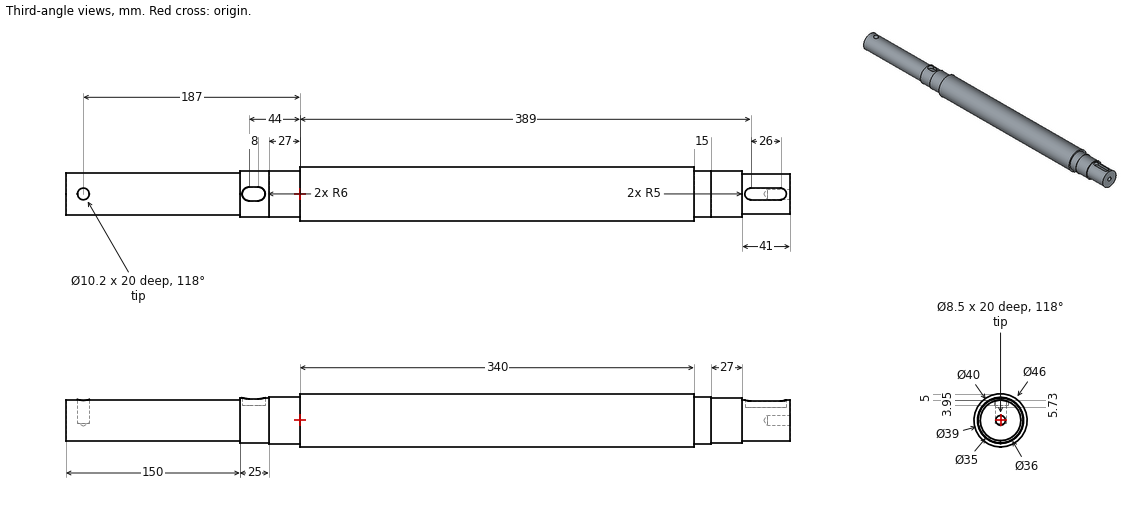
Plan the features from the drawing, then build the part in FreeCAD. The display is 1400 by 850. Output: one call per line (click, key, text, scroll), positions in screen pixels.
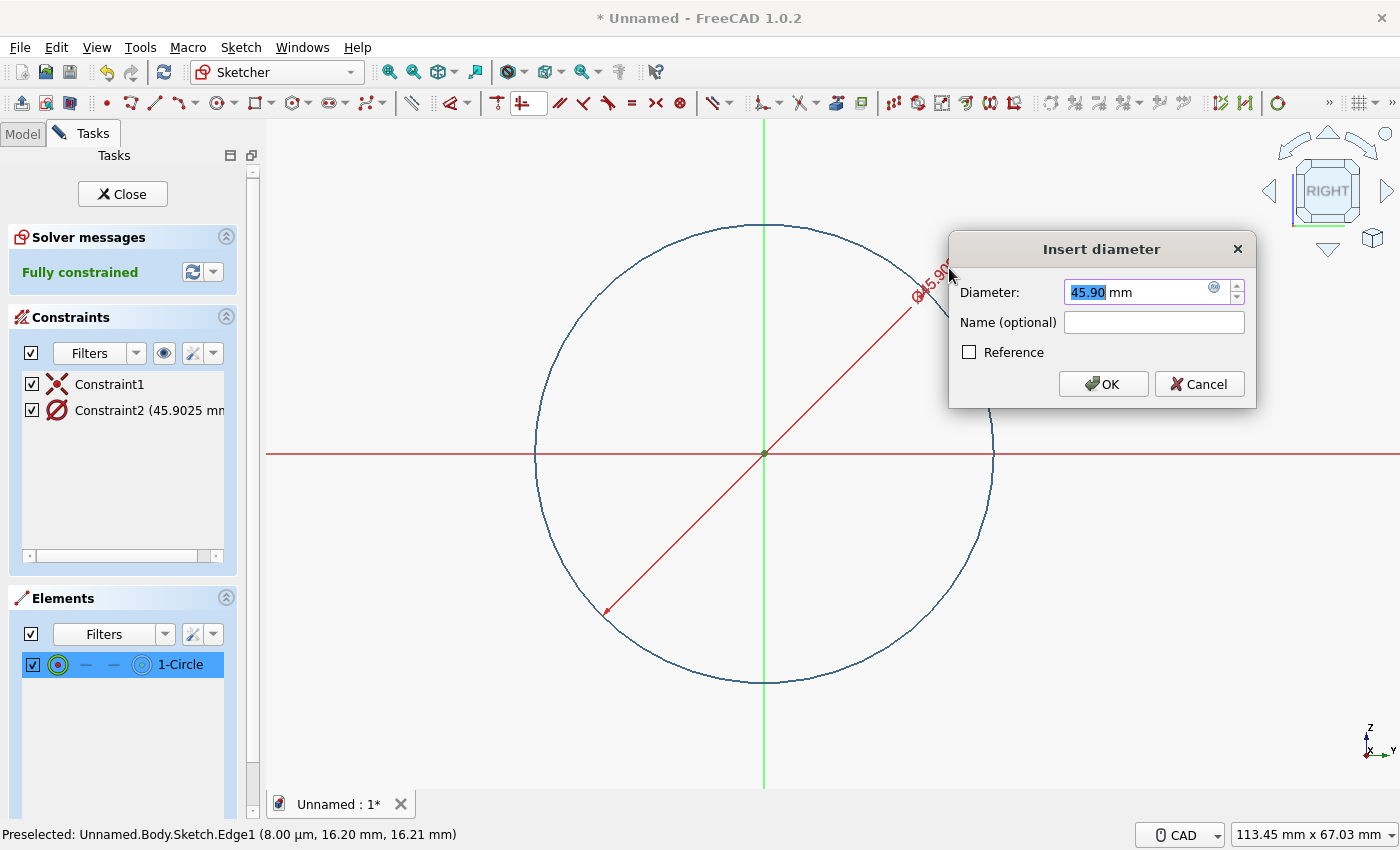
text(46)
key(Return)
key(Escape)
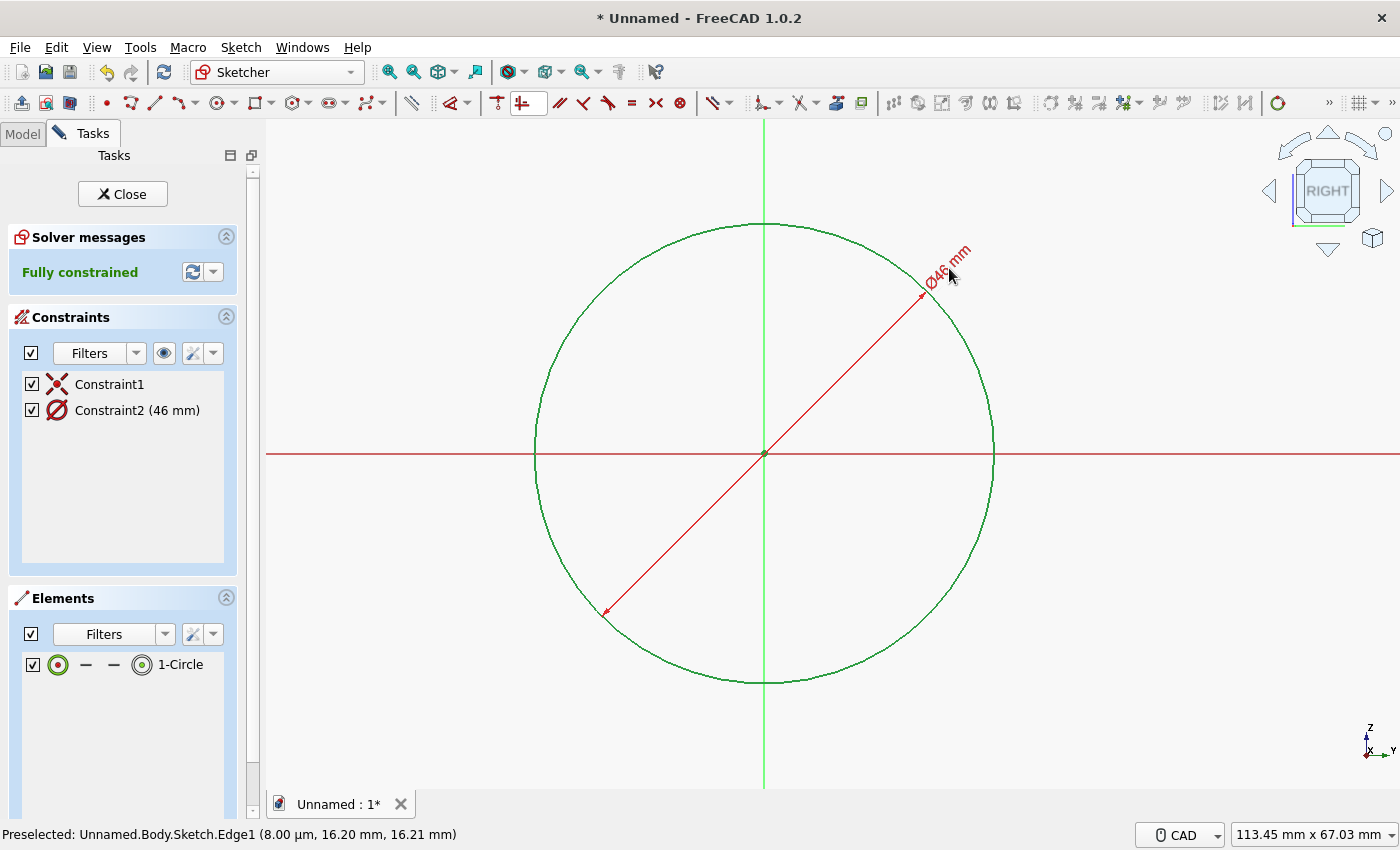
click(123, 194)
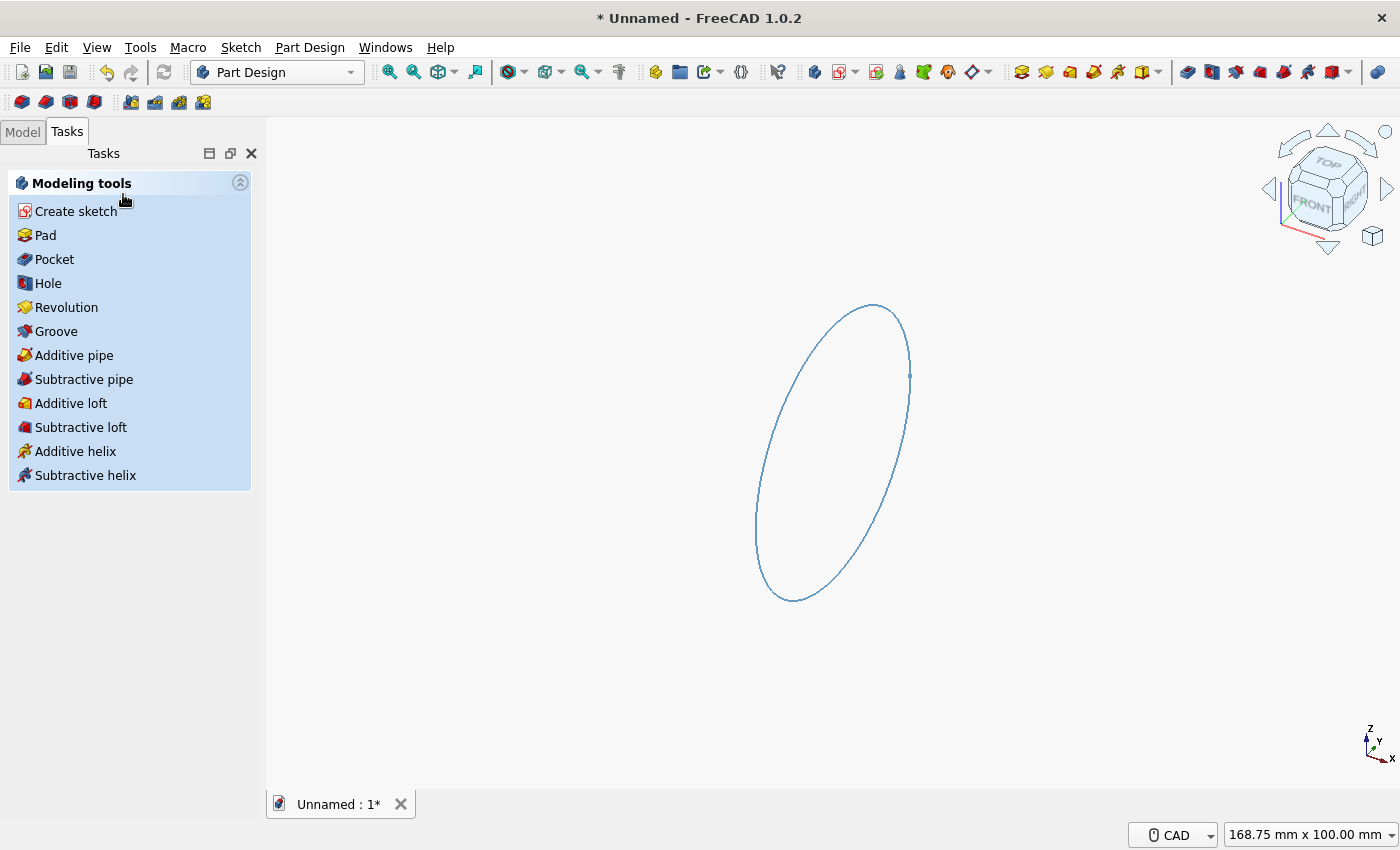
click(1022, 72)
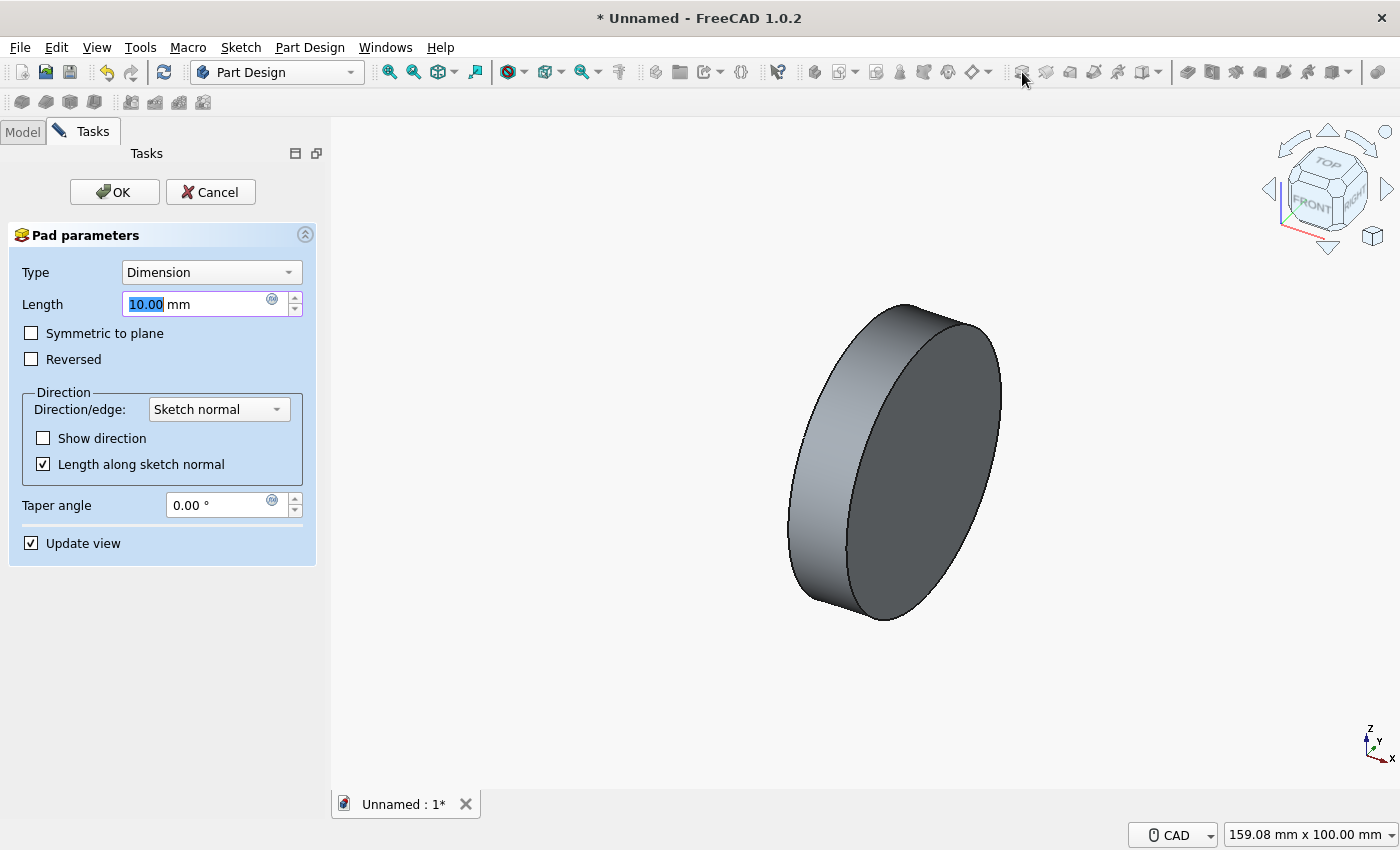
text(340)
key(Tab)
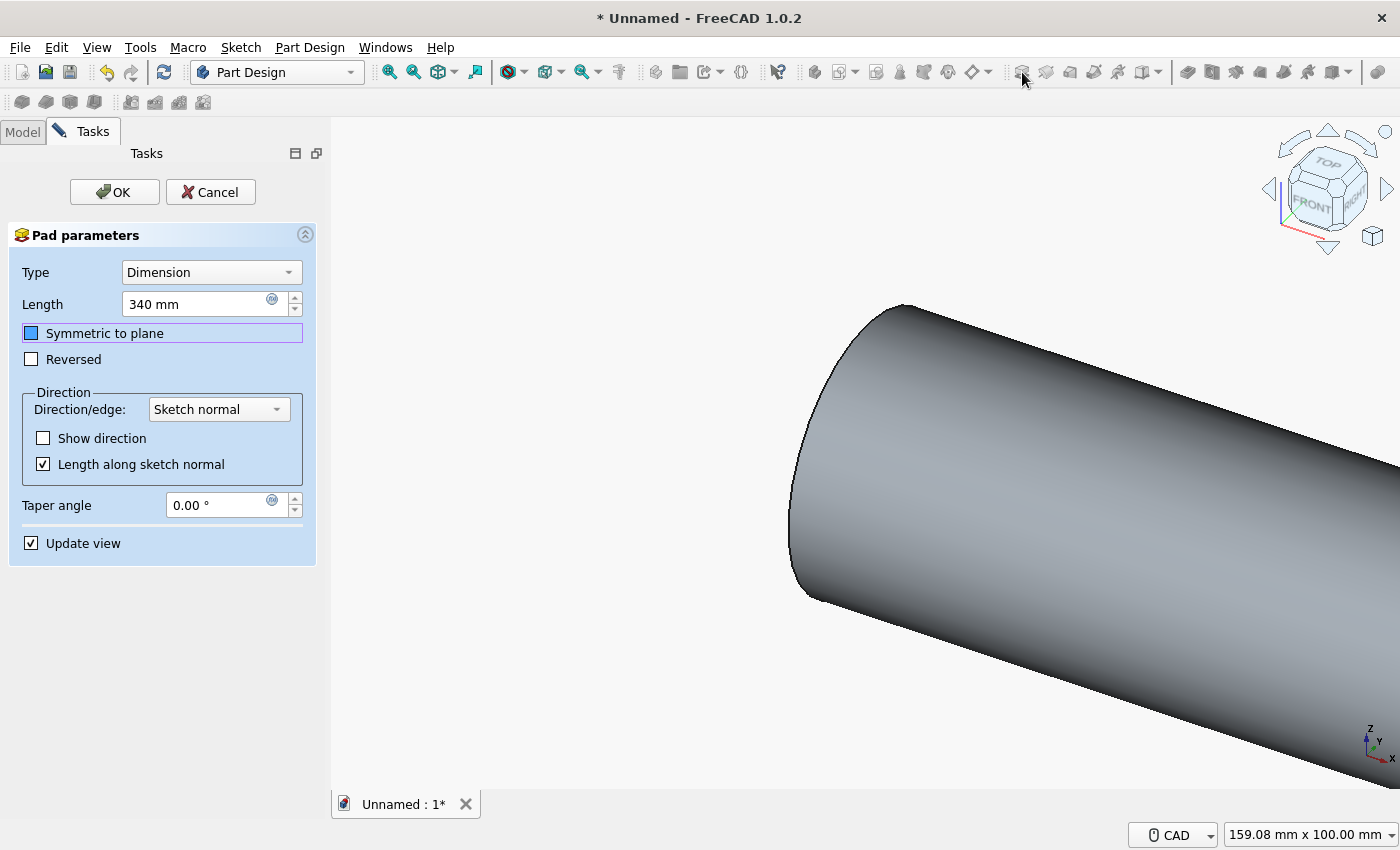
click(115, 192)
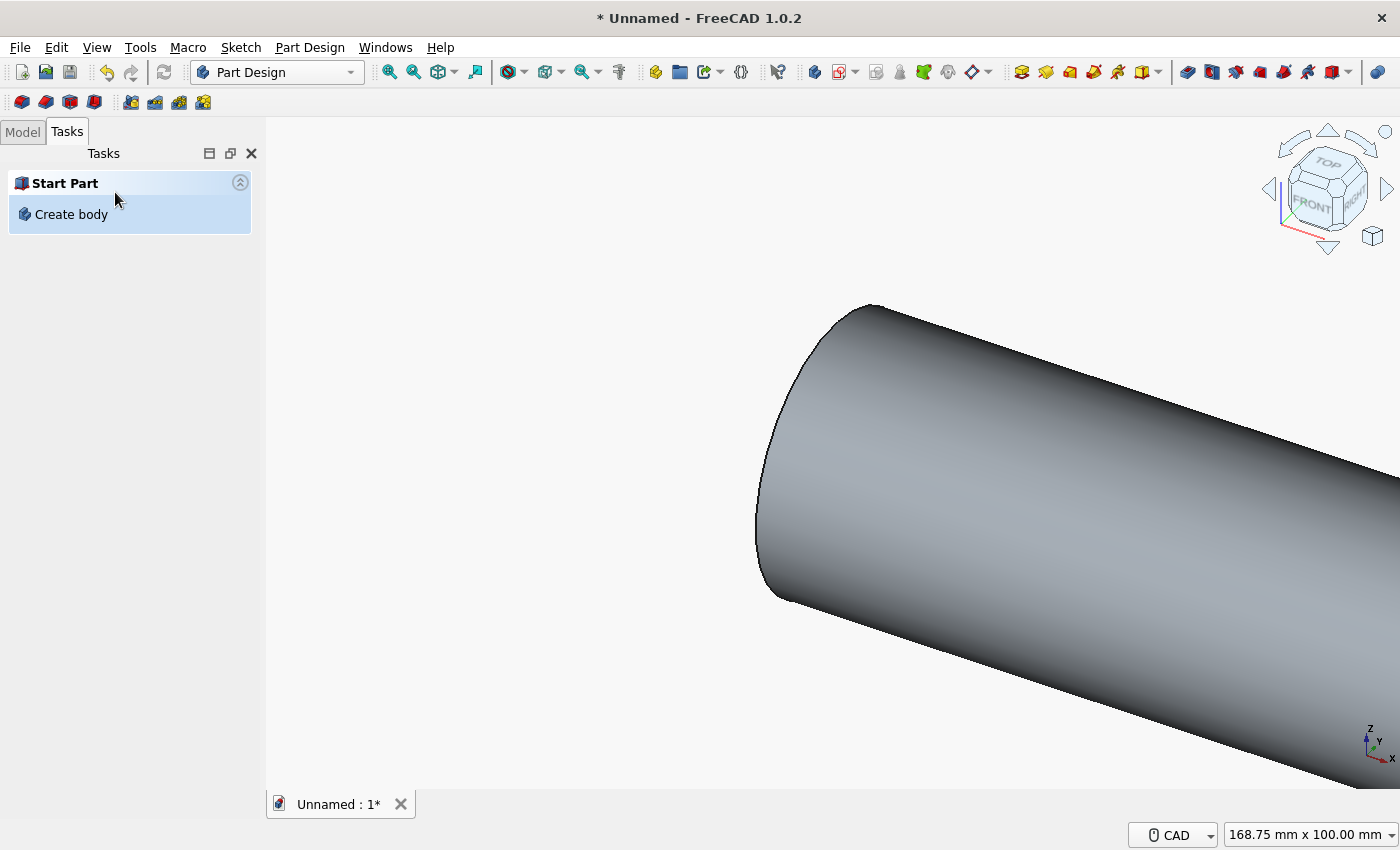
click(390, 72)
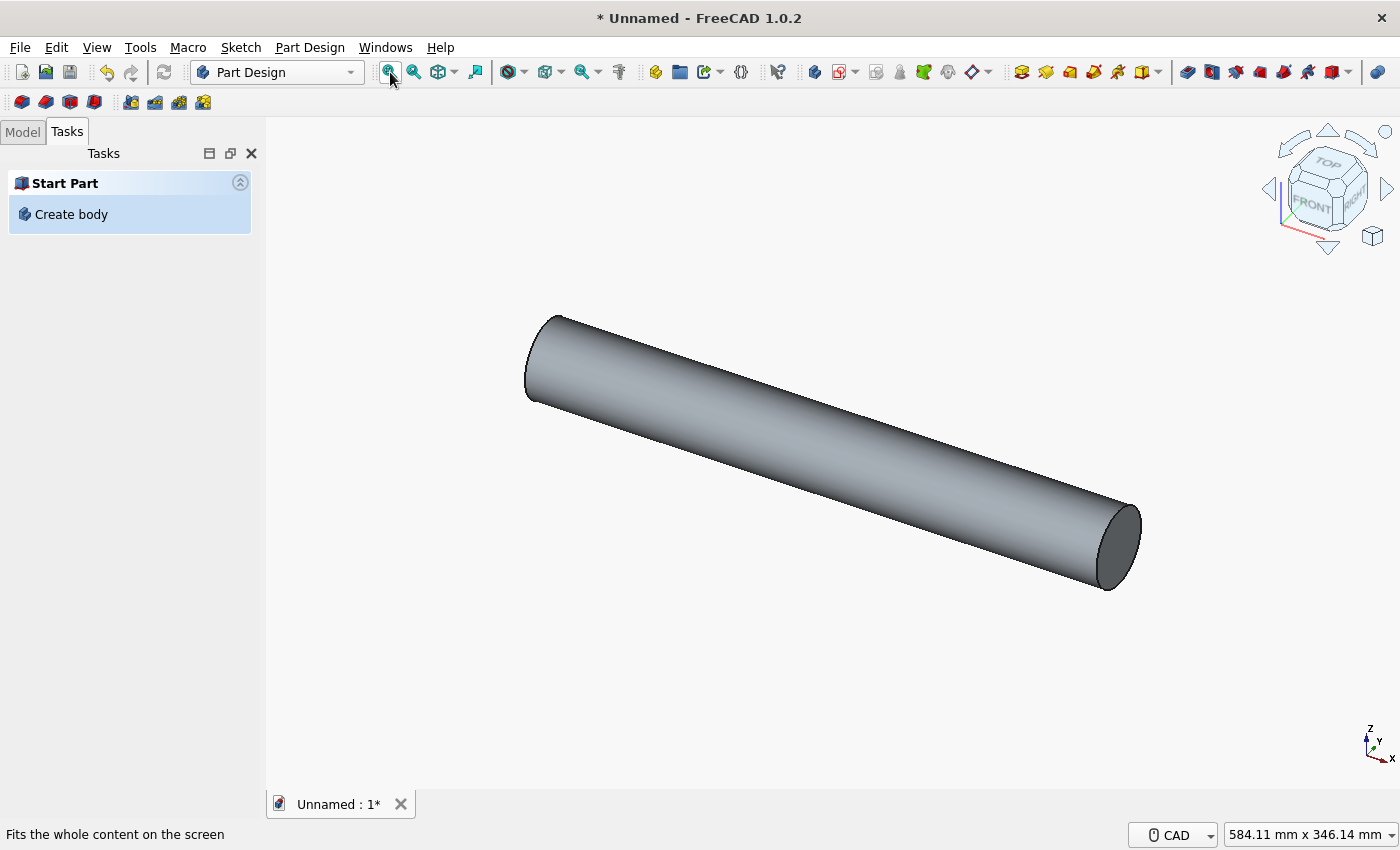
key(6)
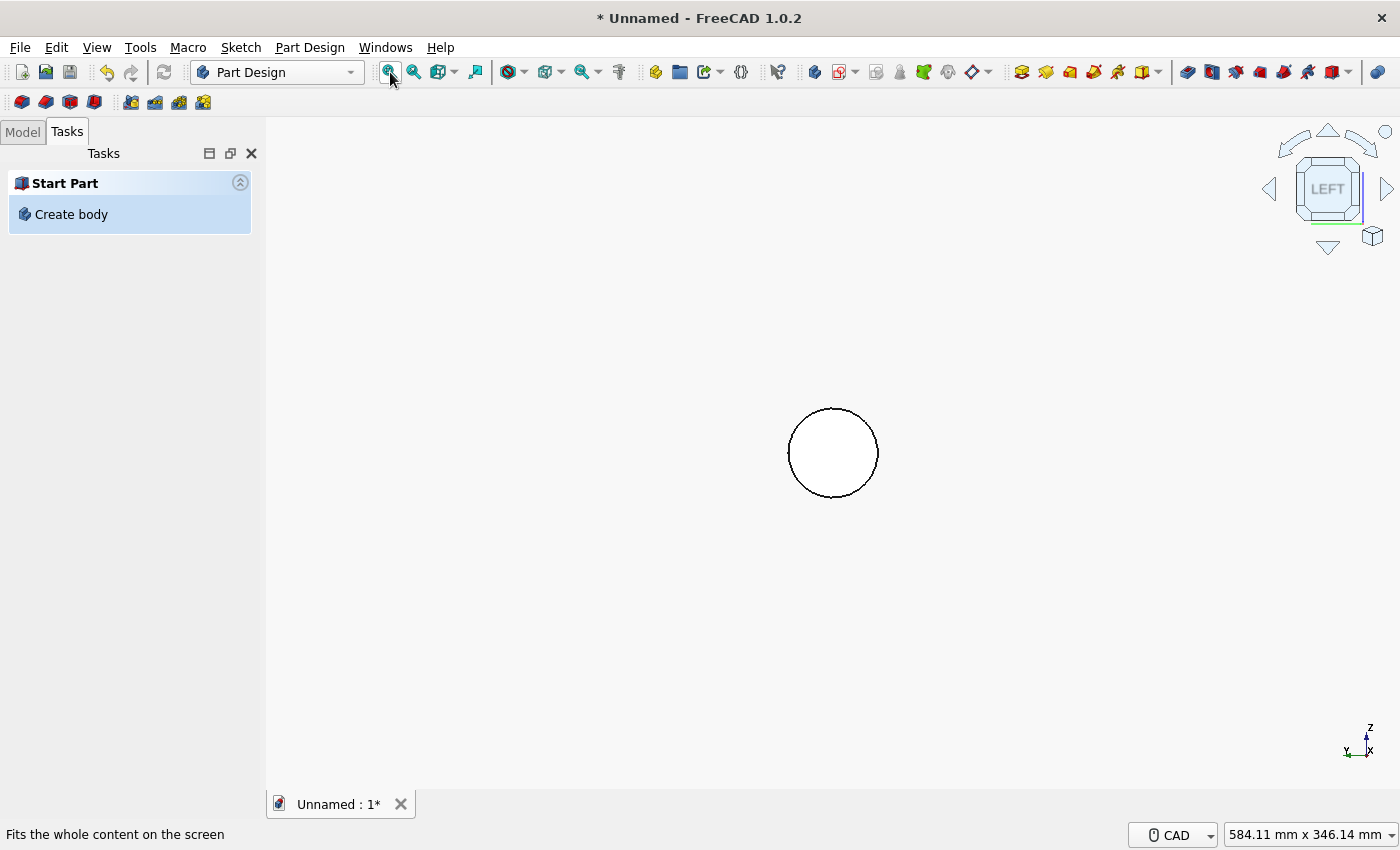
click(390, 72)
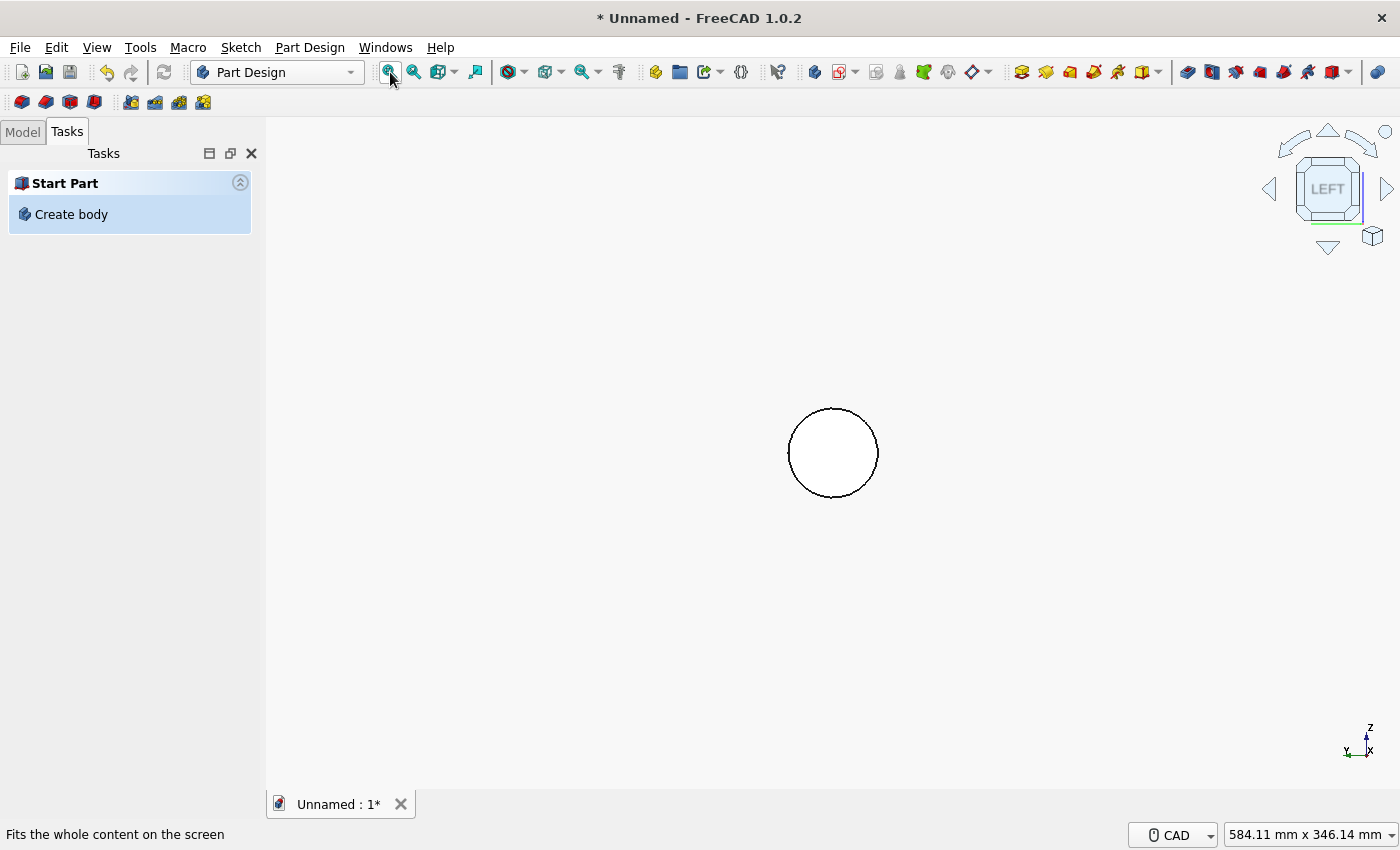
click(833, 452)